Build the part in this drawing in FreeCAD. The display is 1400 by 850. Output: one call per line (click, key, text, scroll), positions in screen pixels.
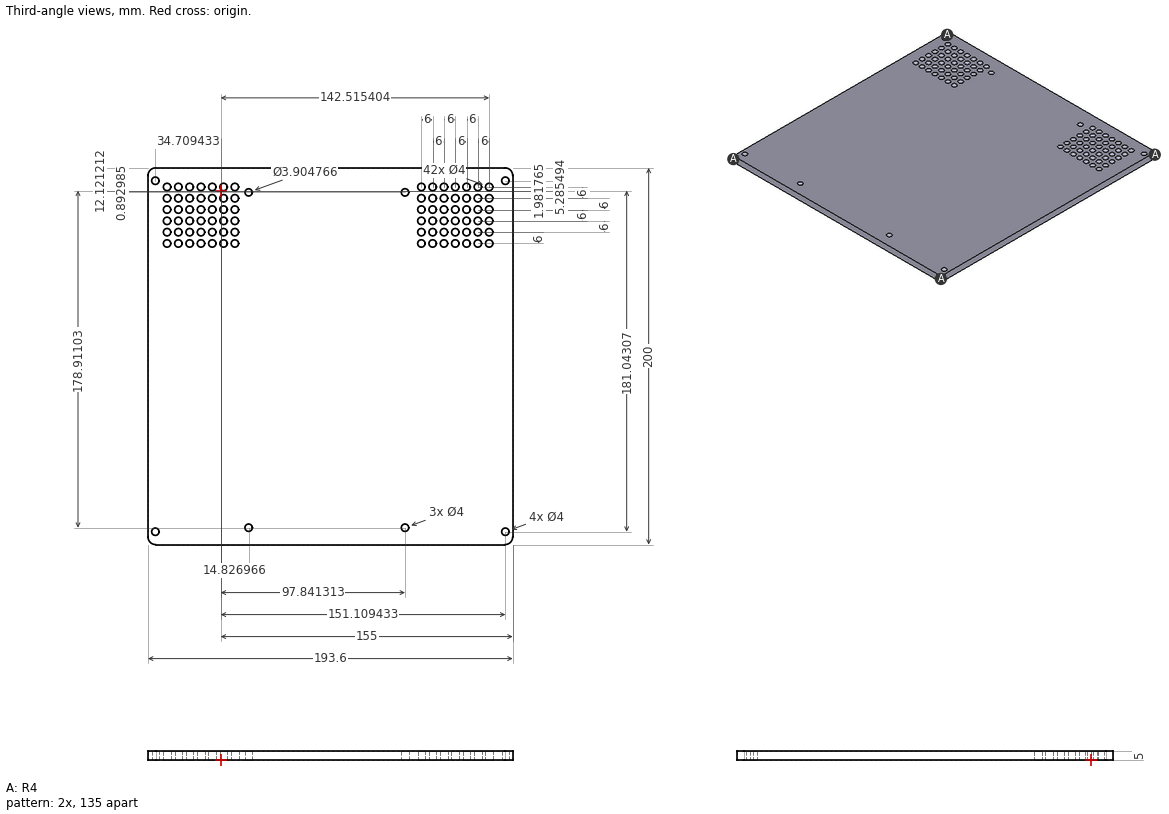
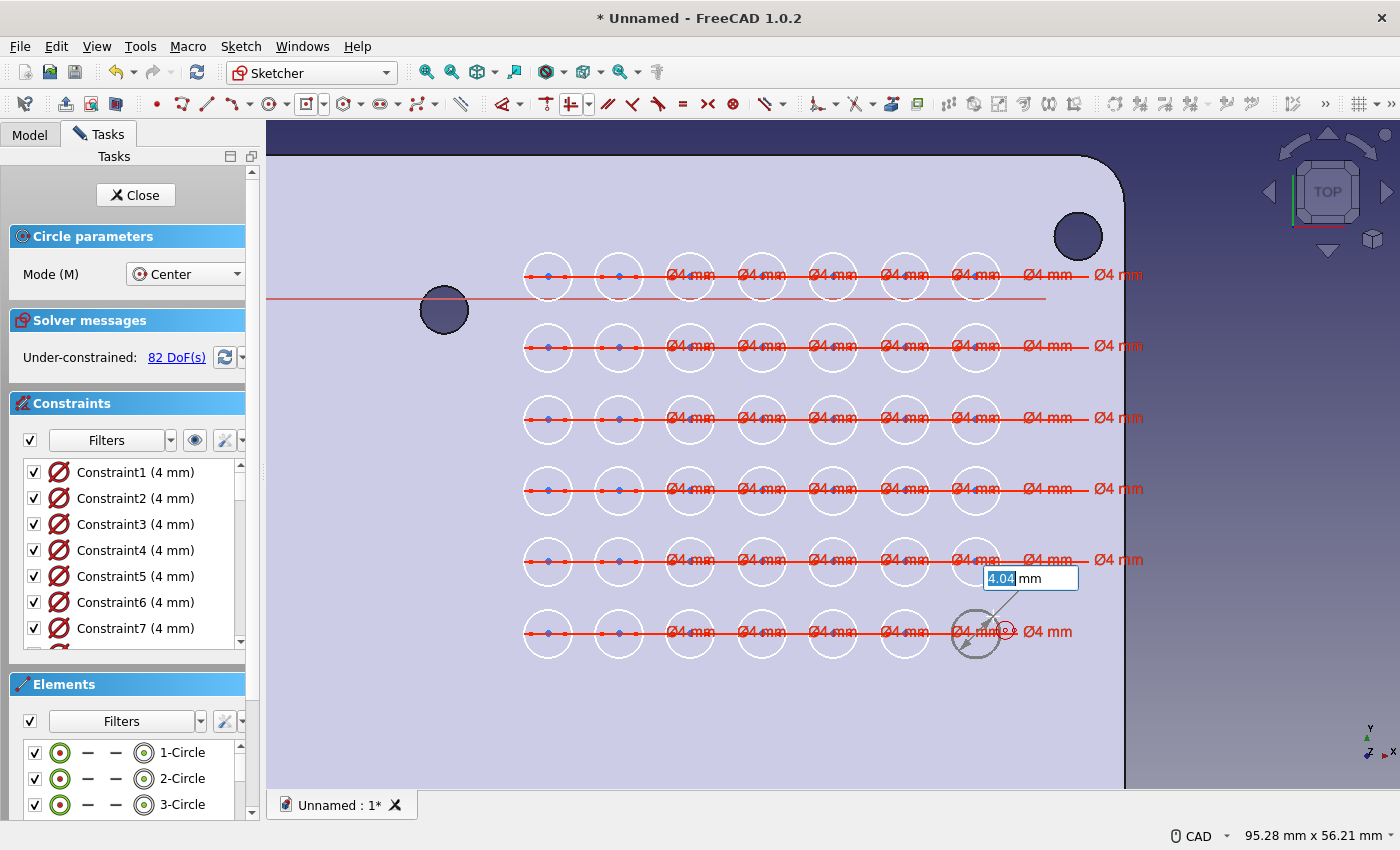
text(4)
key(Return)
key(Escape)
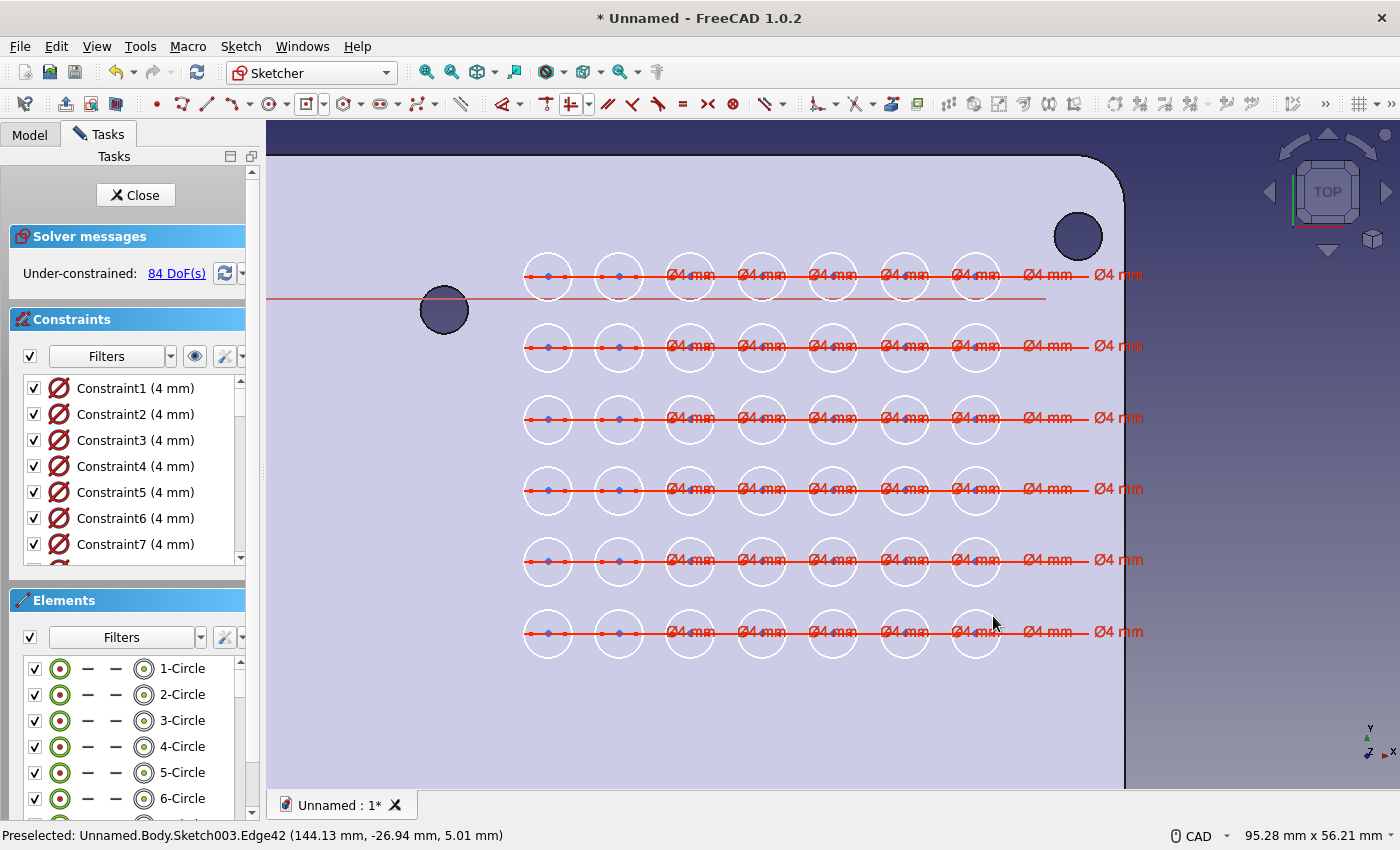
click(502, 104)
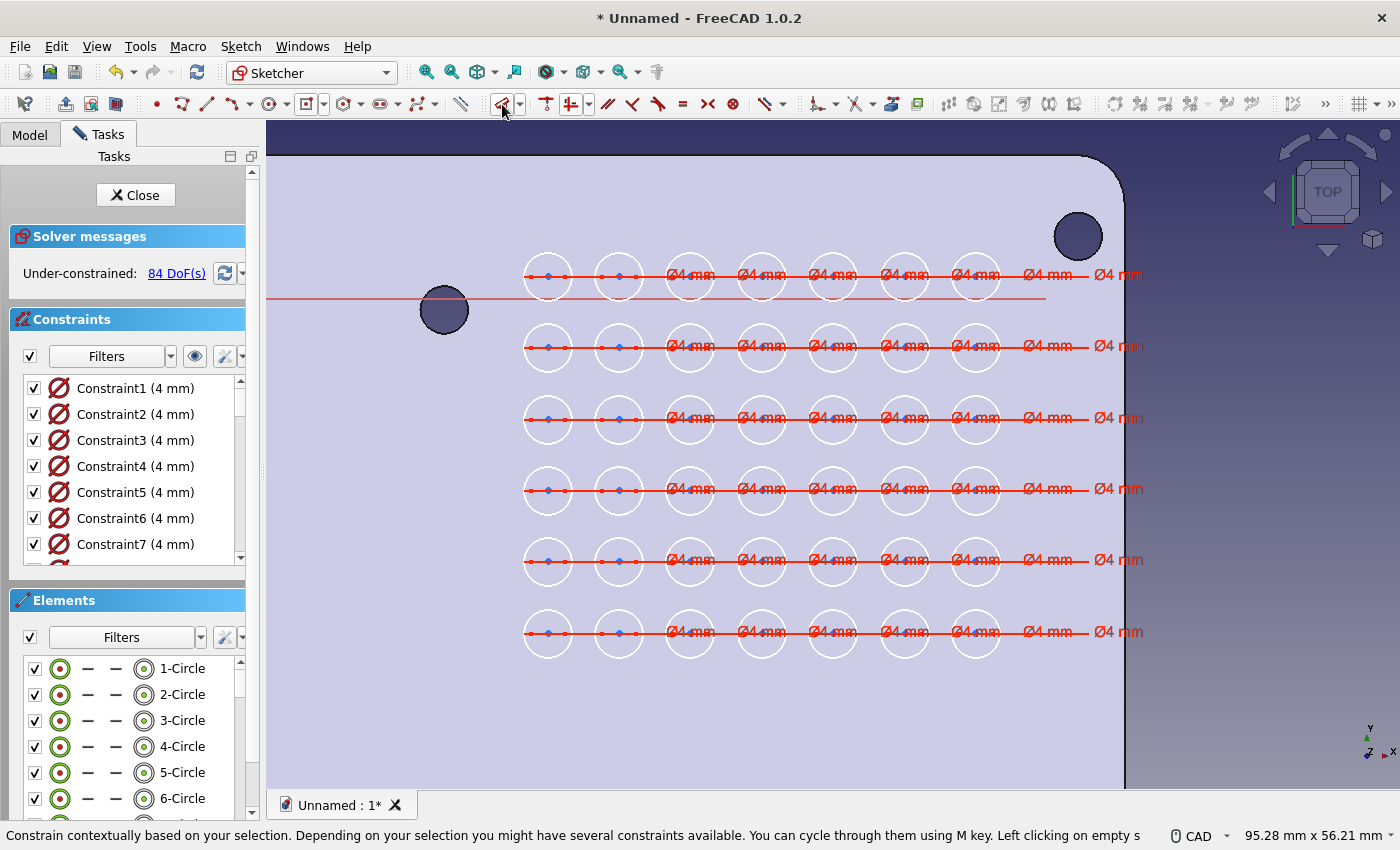
click(976, 277)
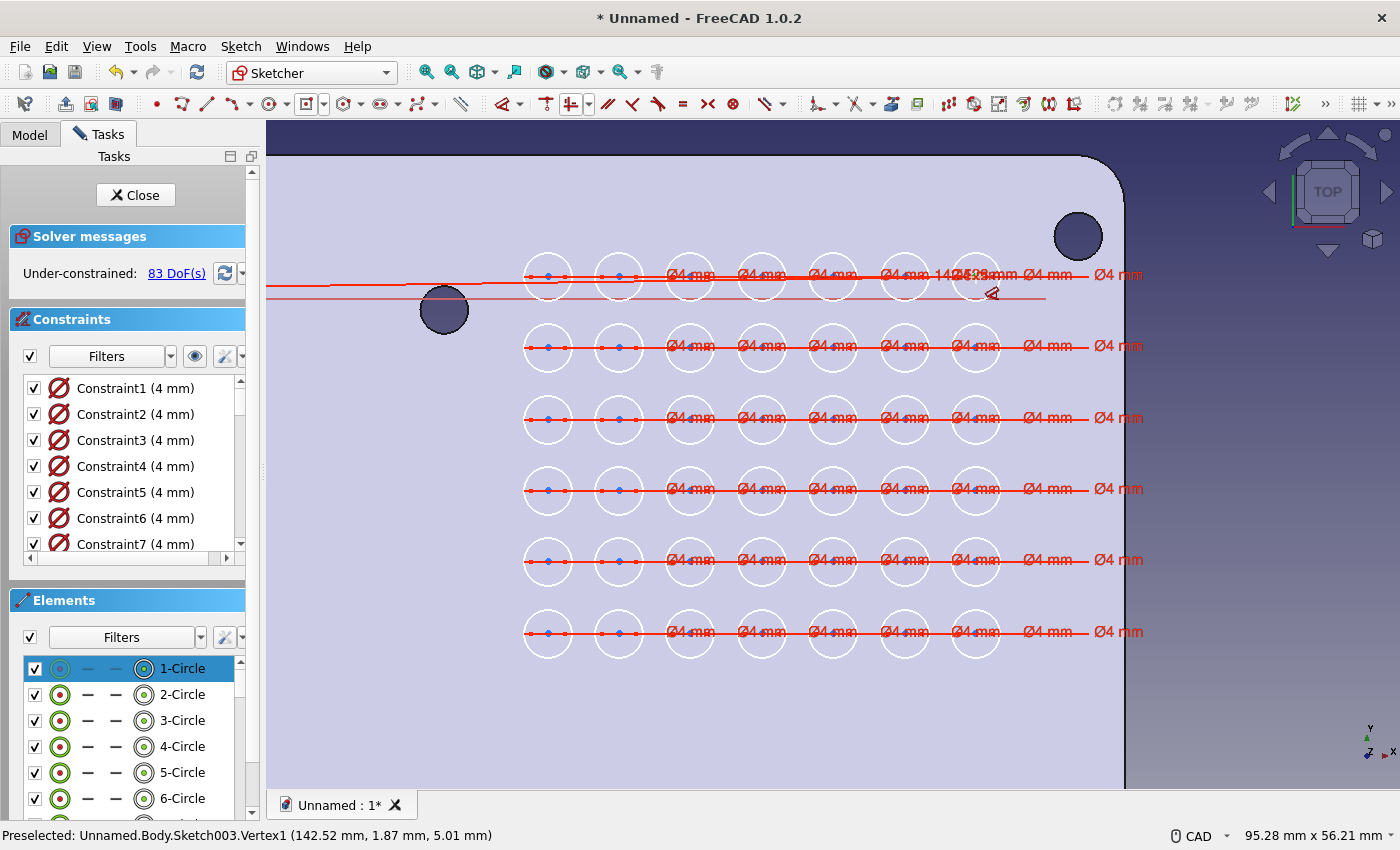
click(905, 277)
click(940, 243)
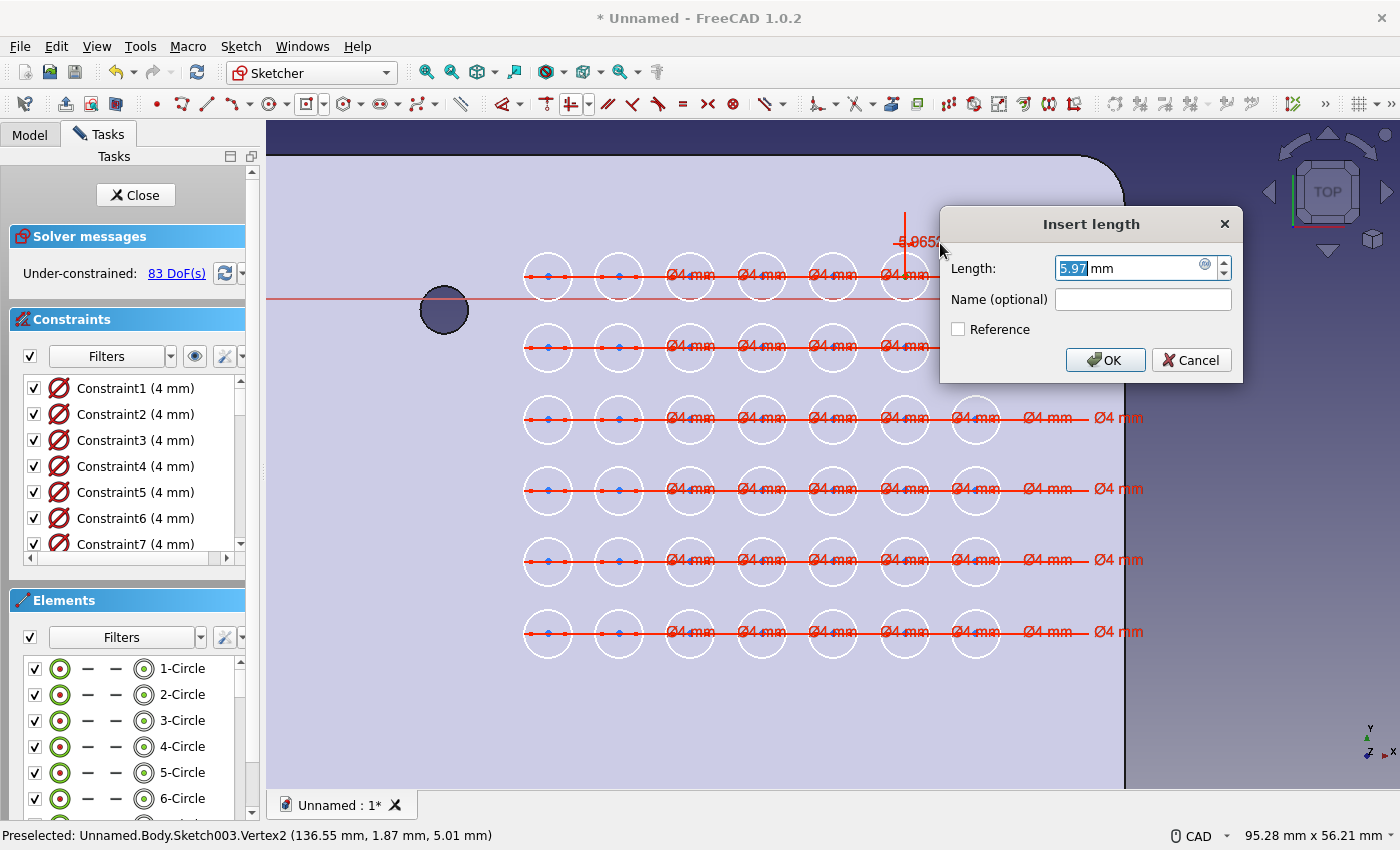
text(6)
key(Return)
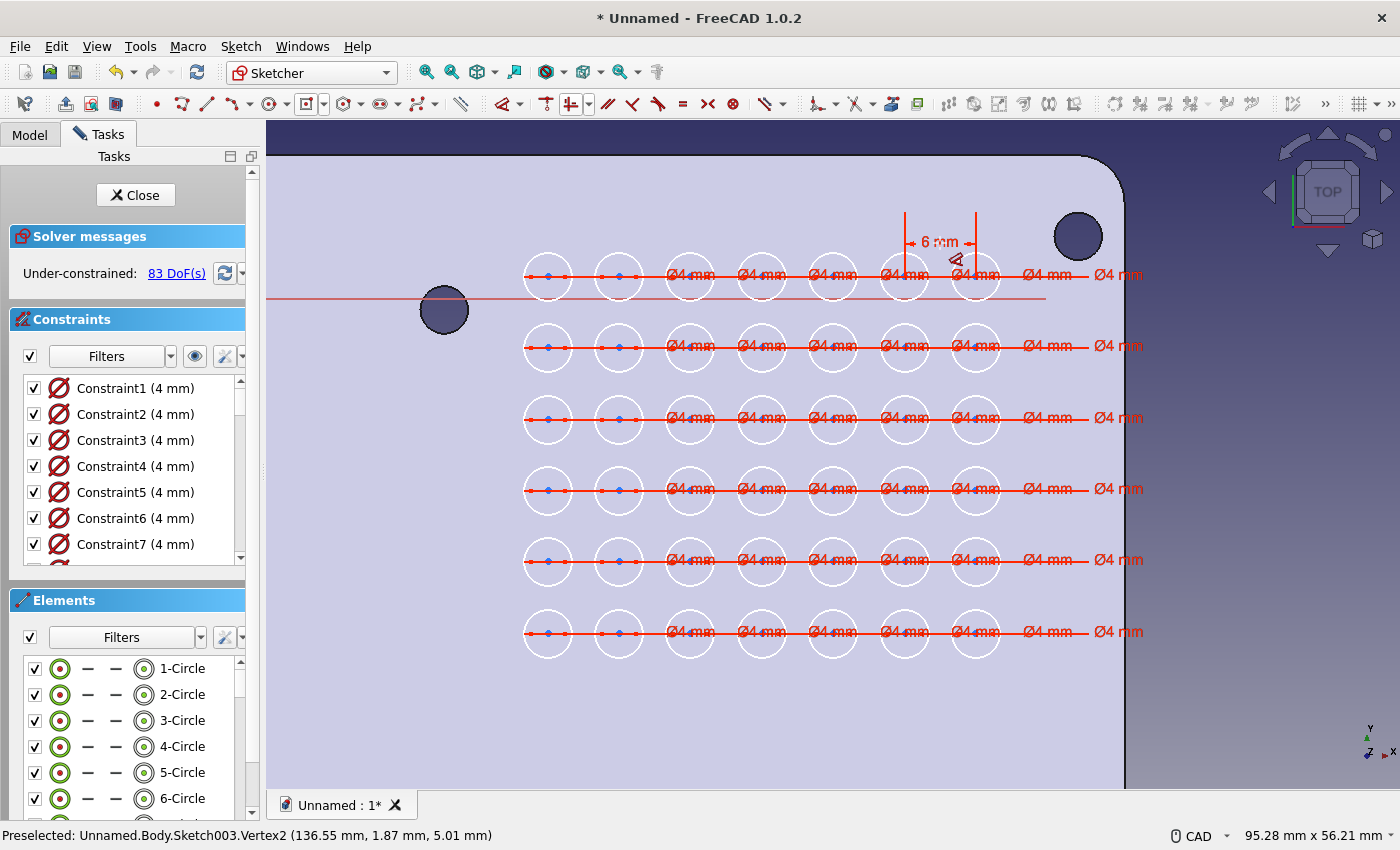
click(905, 277)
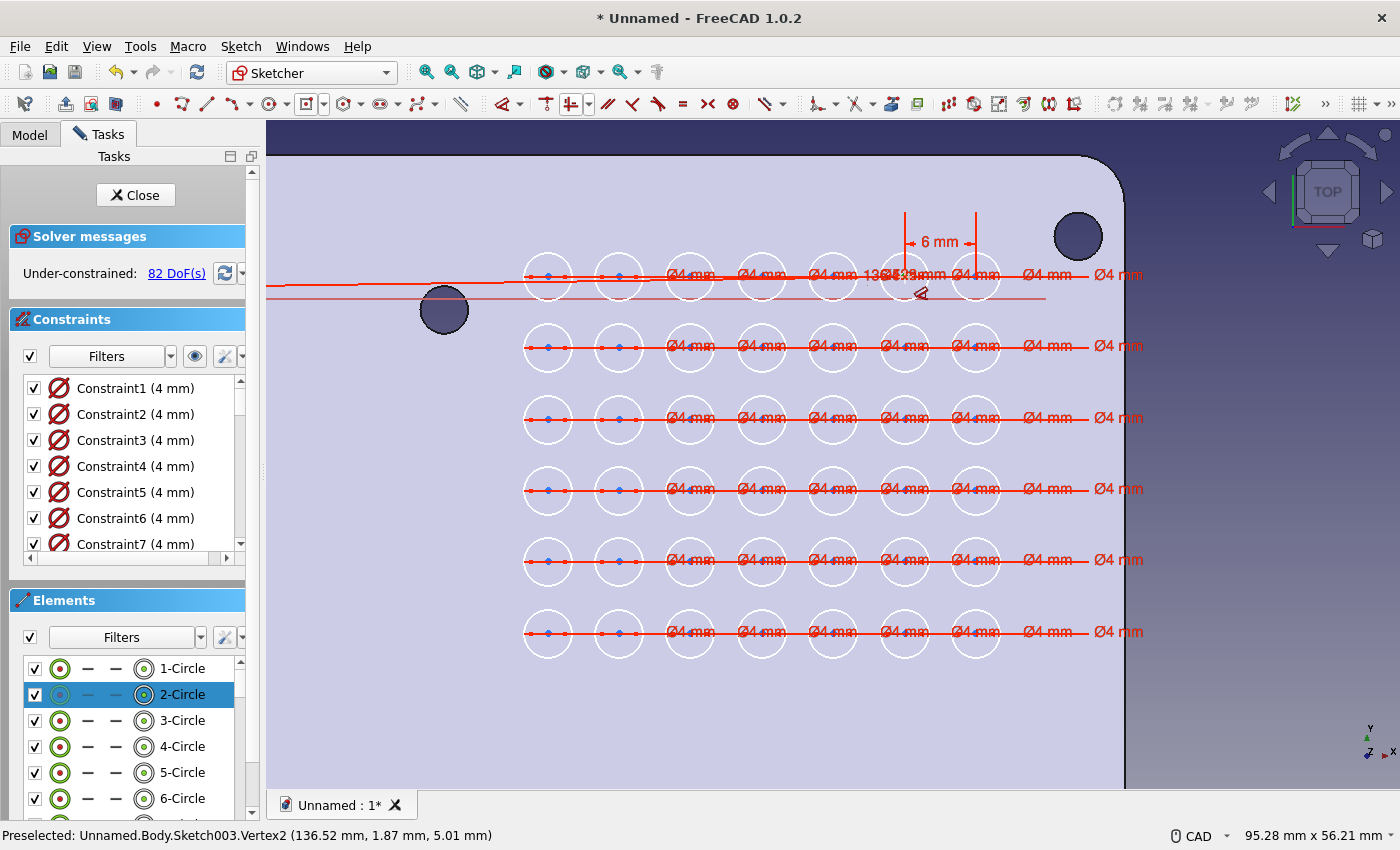
click(833, 277)
click(869, 243)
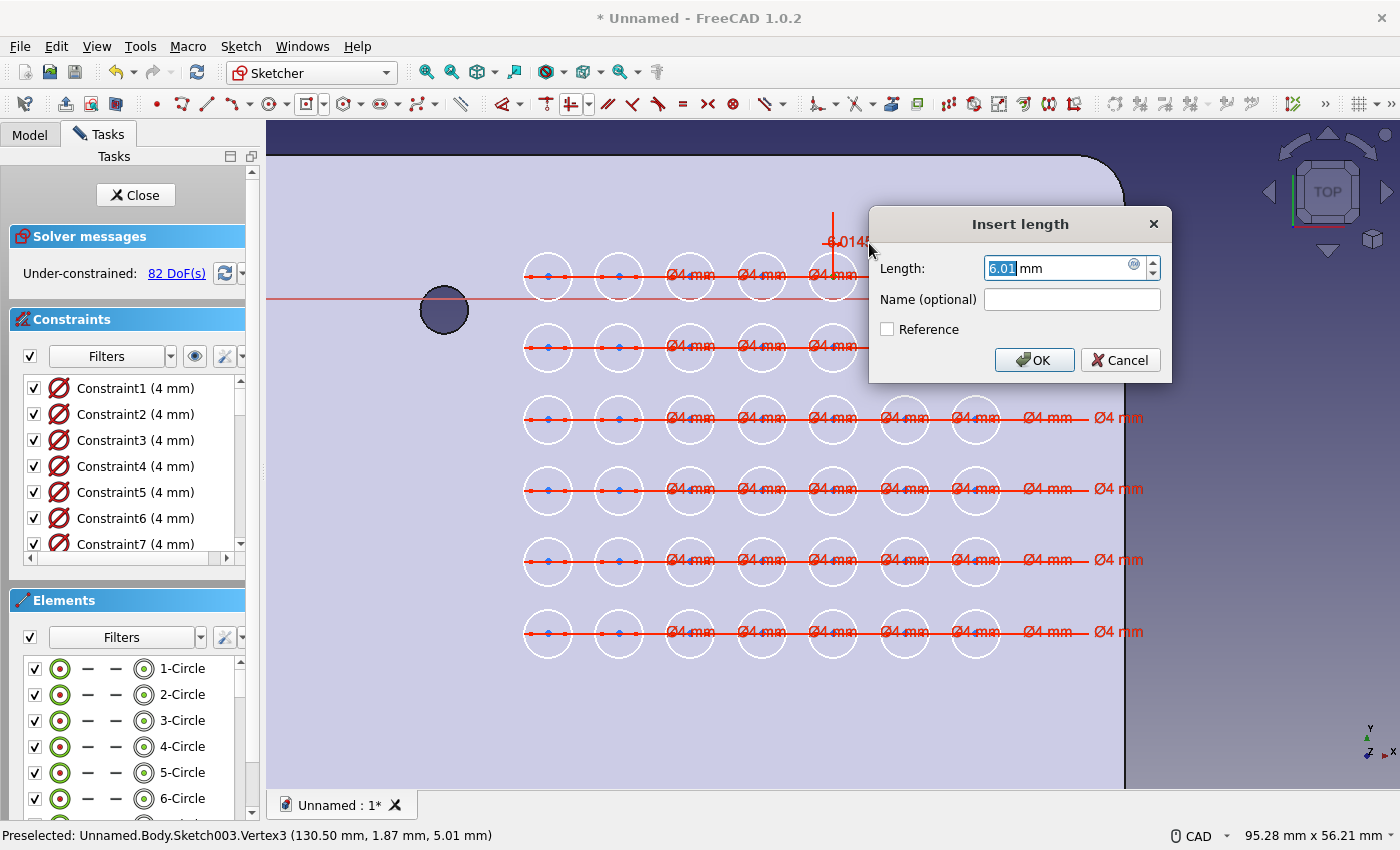
text(6)
key(Return)